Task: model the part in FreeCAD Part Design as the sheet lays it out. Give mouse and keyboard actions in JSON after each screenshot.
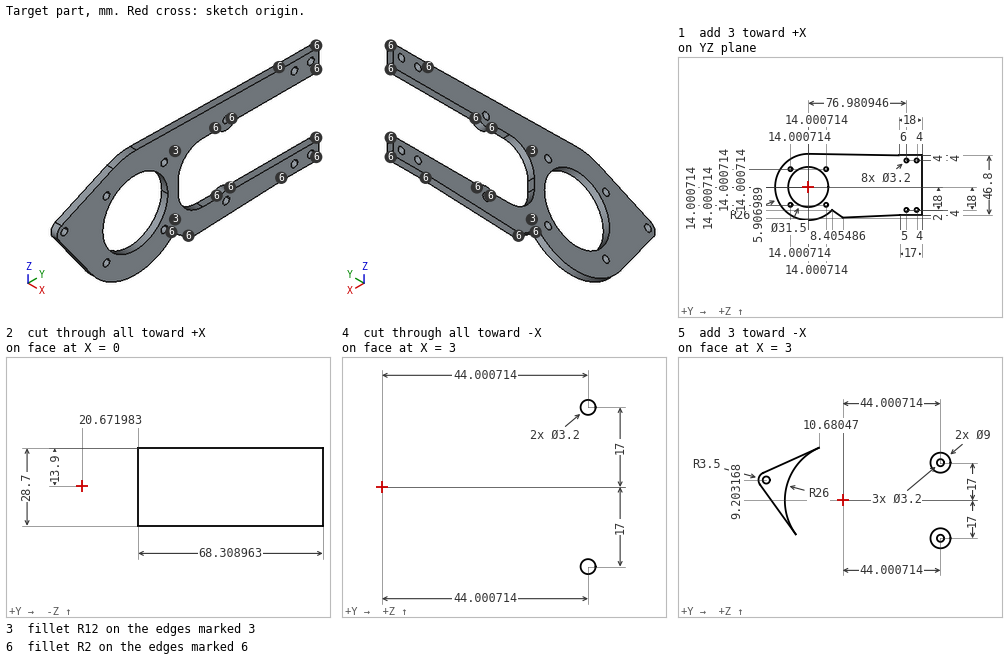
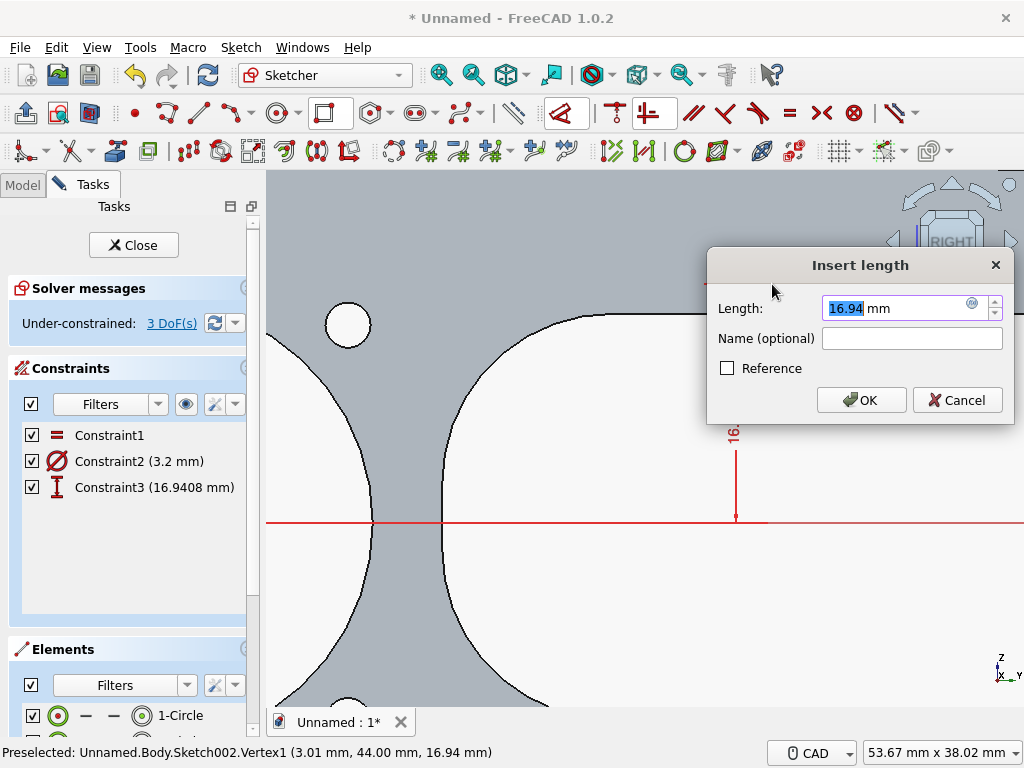
{"action": "type", "text": "17"}
{"action": "key", "text": "Return"}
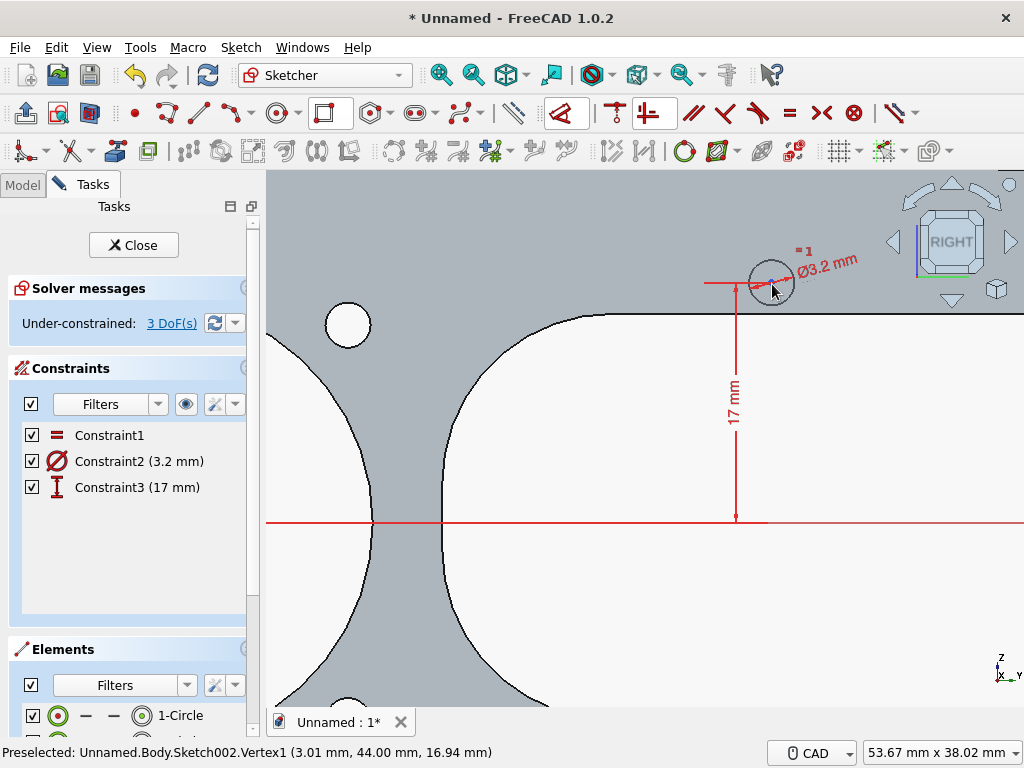
{"action": "scroll", "coordinate": [788, 267], "scroll_direction": "down", "scroll_amount": 2}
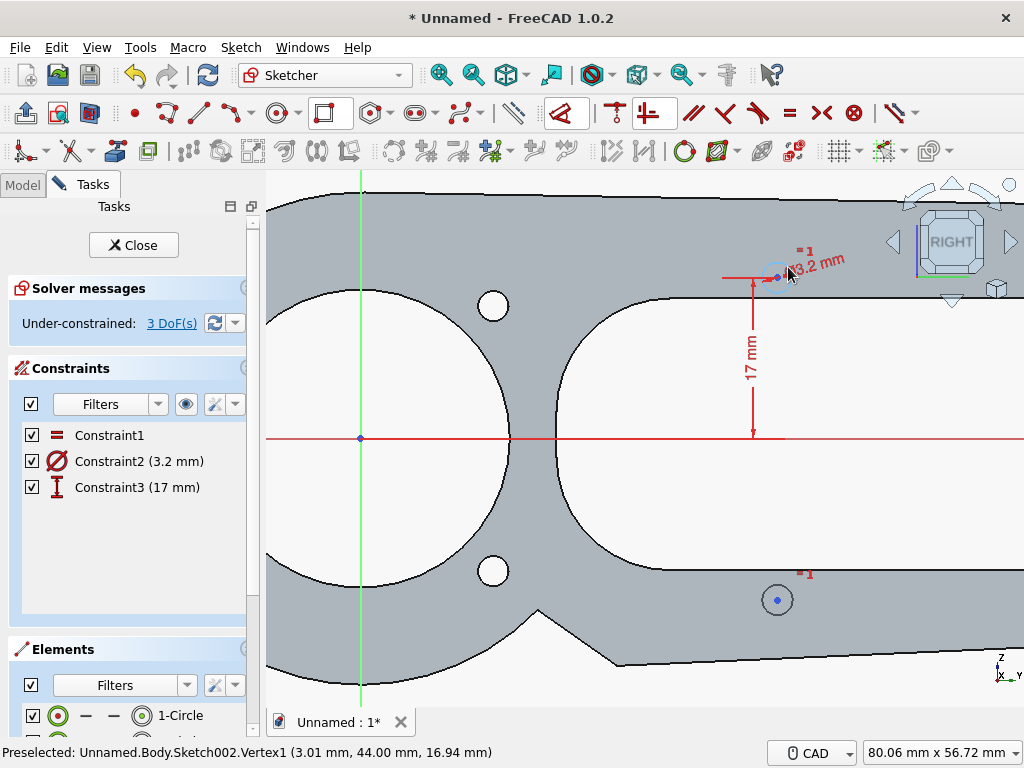
{"action": "left_click", "coordinate": [777, 600]}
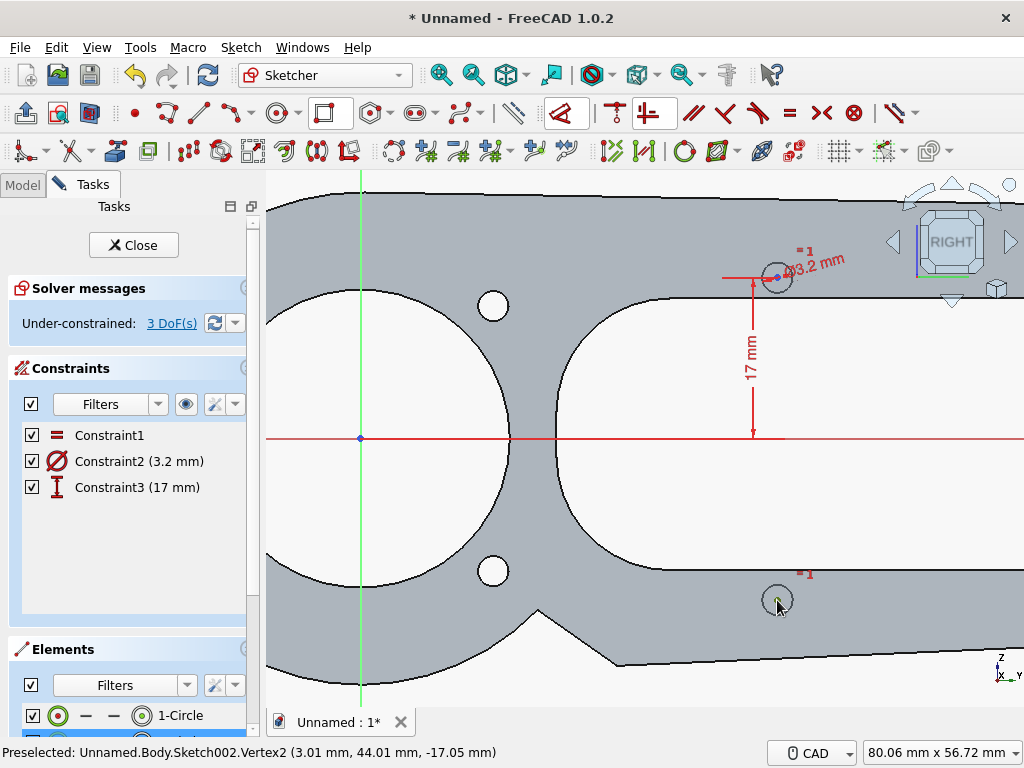
{"action": "left_click", "coordinate": [584, 114]}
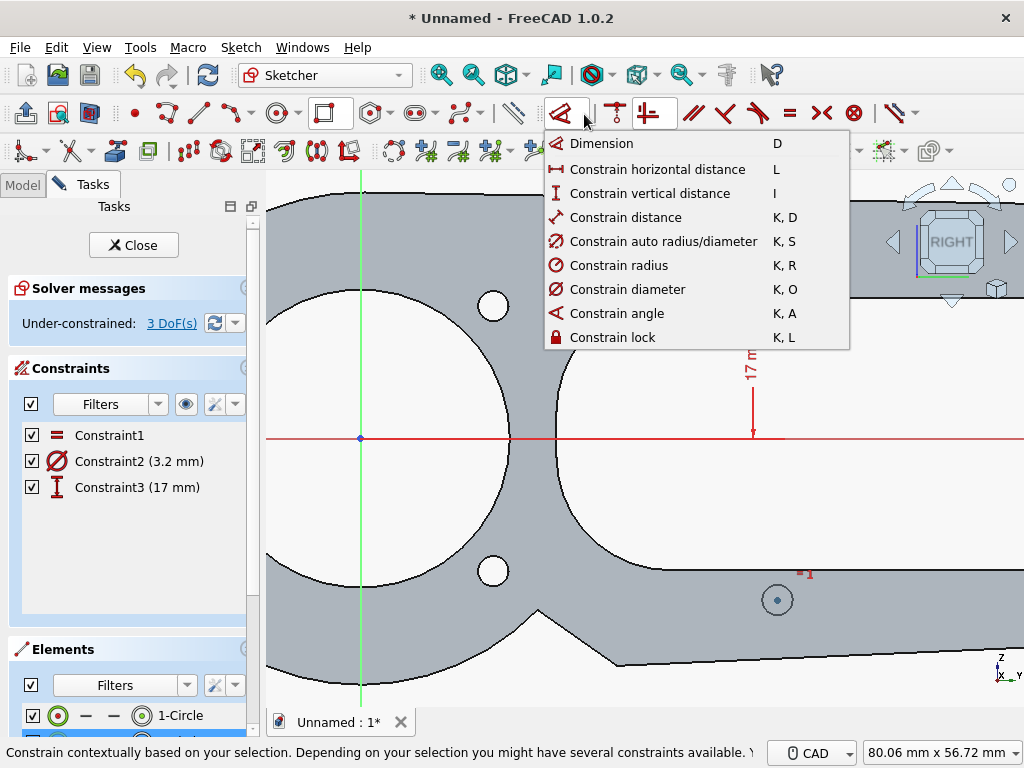
{"action": "left_click", "coordinate": [697, 193]}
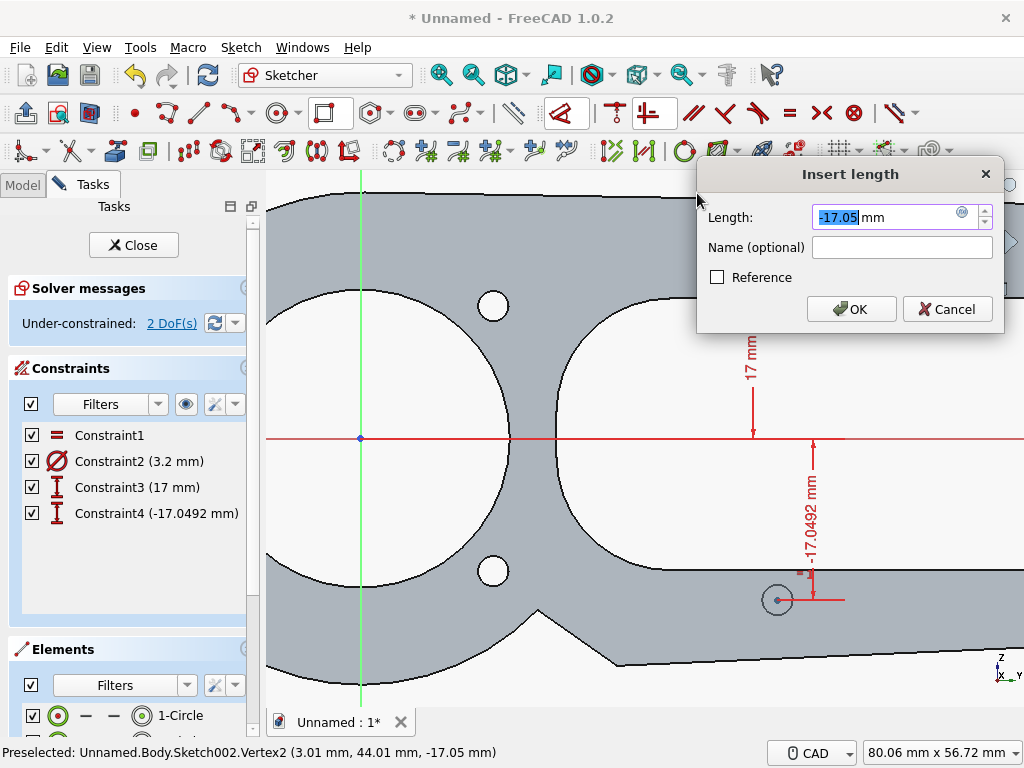
{"action": "type", "text": "-17"}
{"action": "key", "text": "Return"}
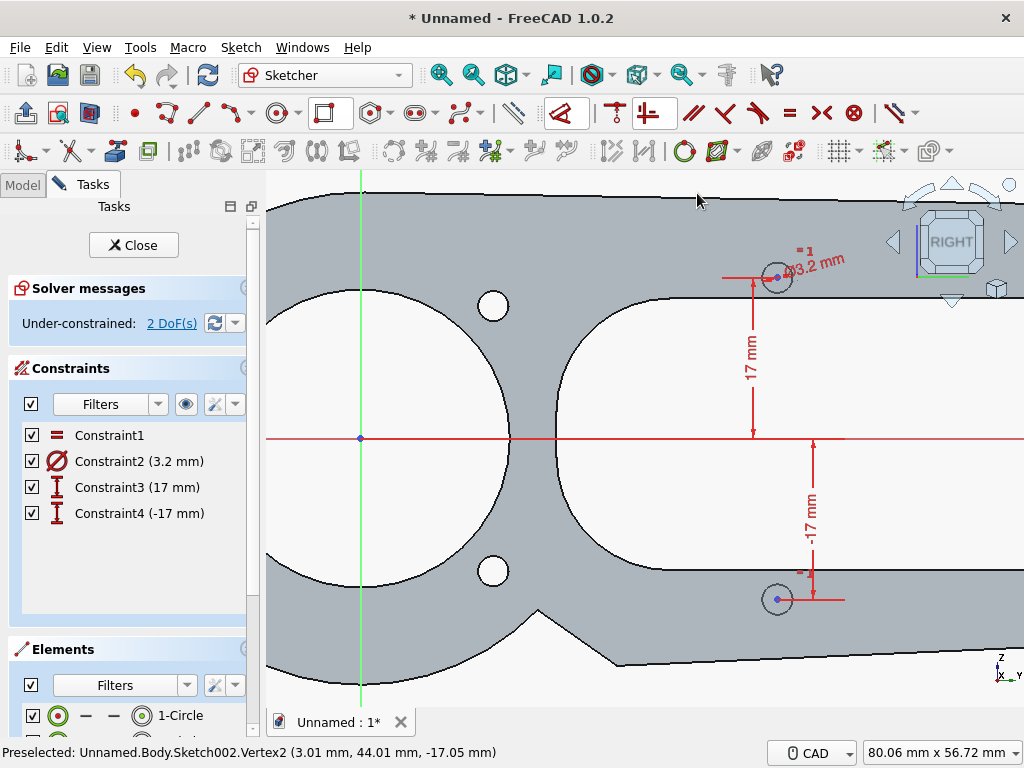
{"action": "left_click", "coordinate": [777, 278]}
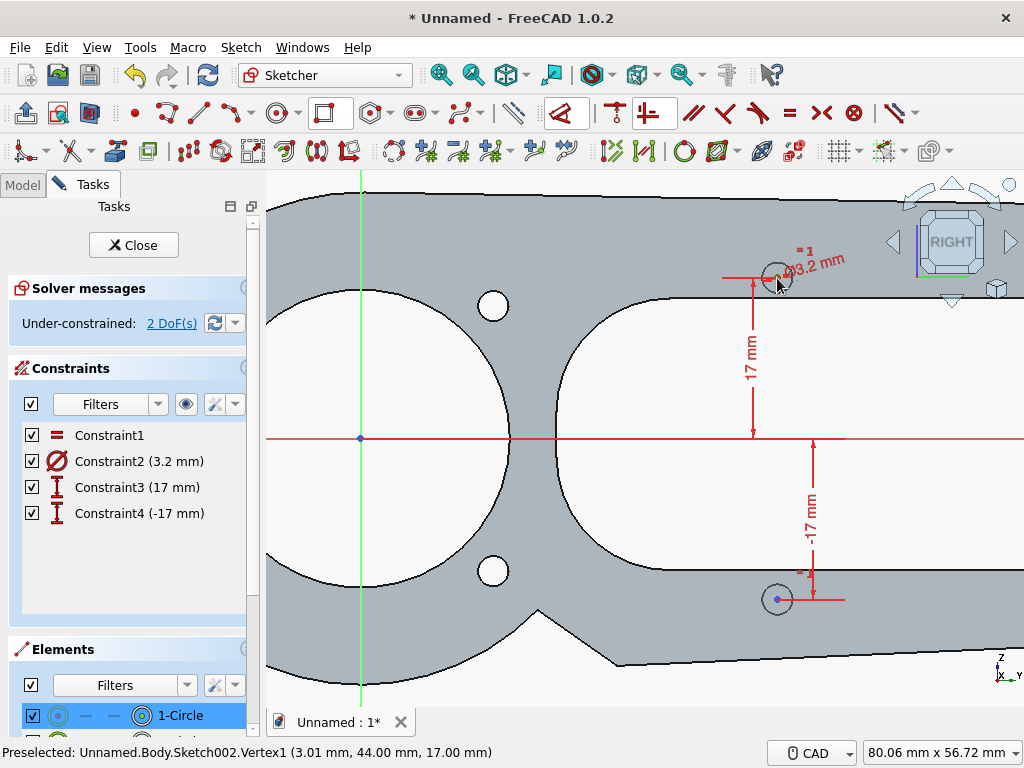
{"action": "key", "text": "l"}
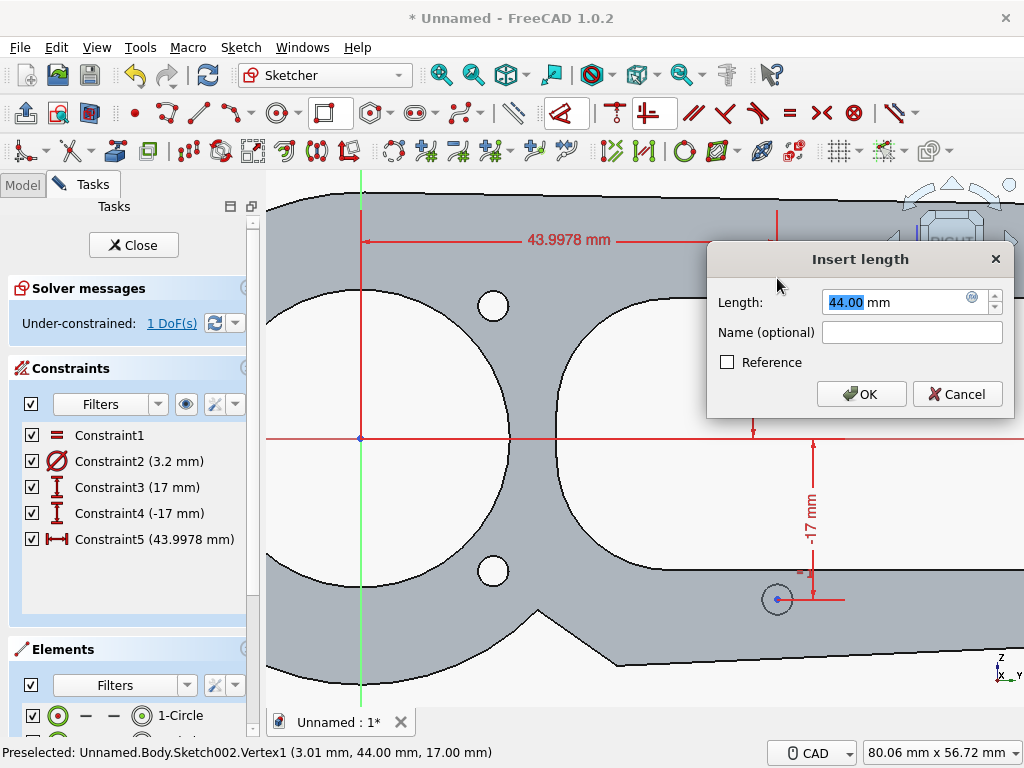
{"action": "type", "text": "44.000714"}
{"action": "key", "text": "Return"}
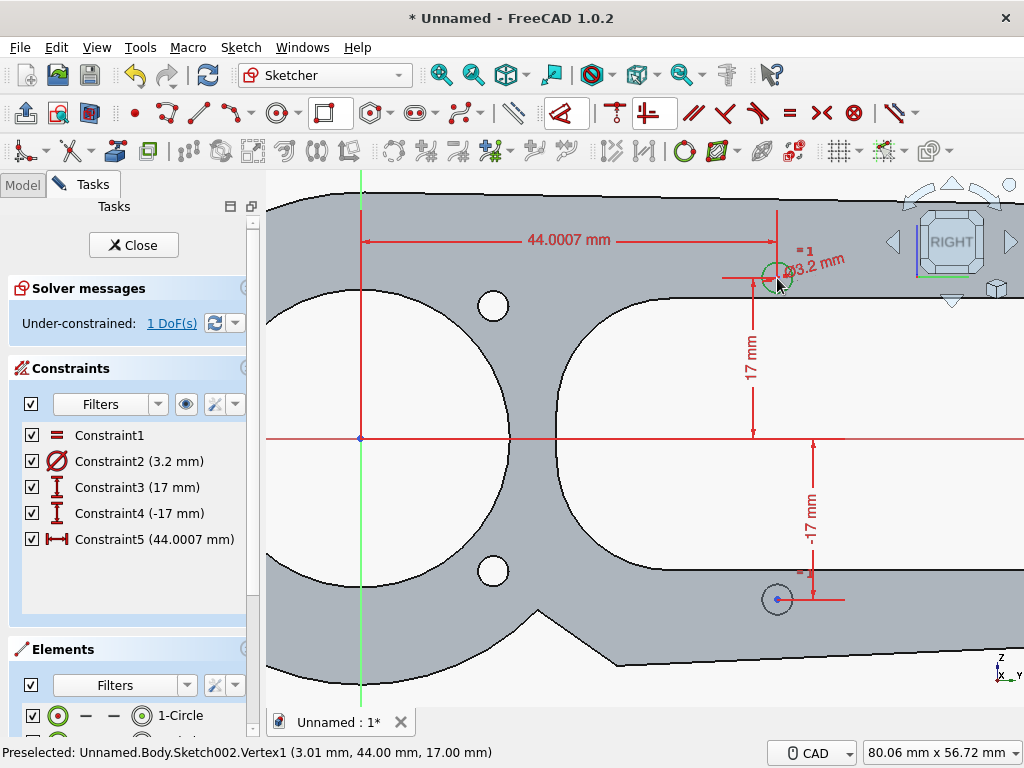
{"action": "left_click", "coordinate": [777, 600]}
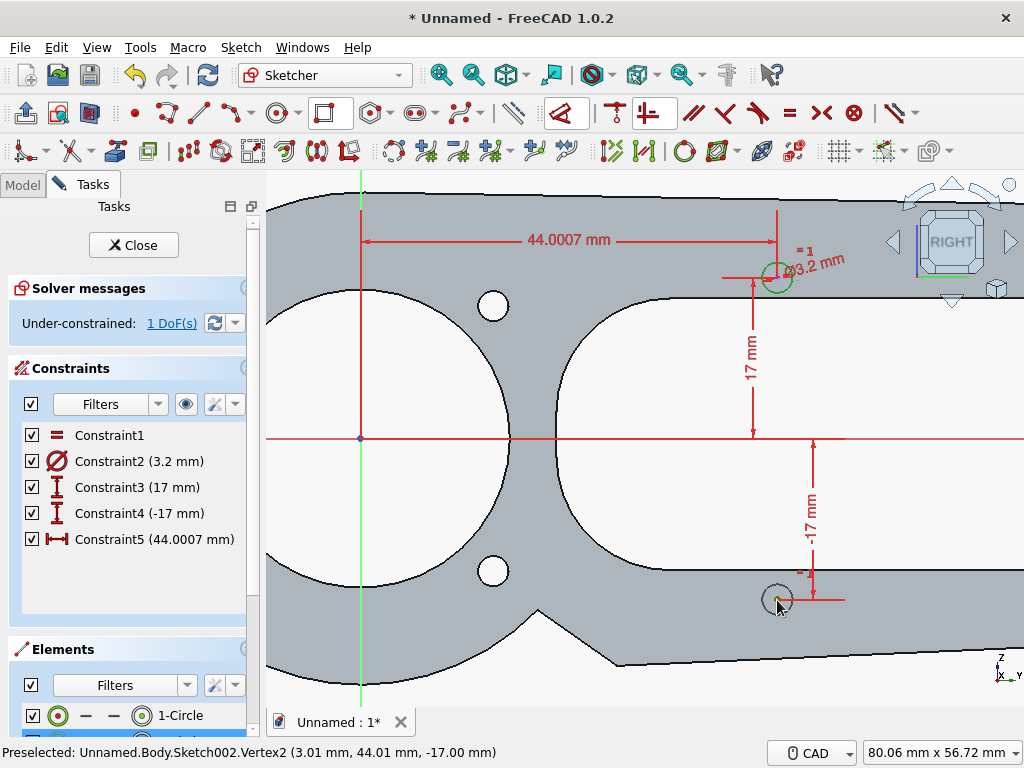
{"action": "left_click", "coordinate": [584, 114]}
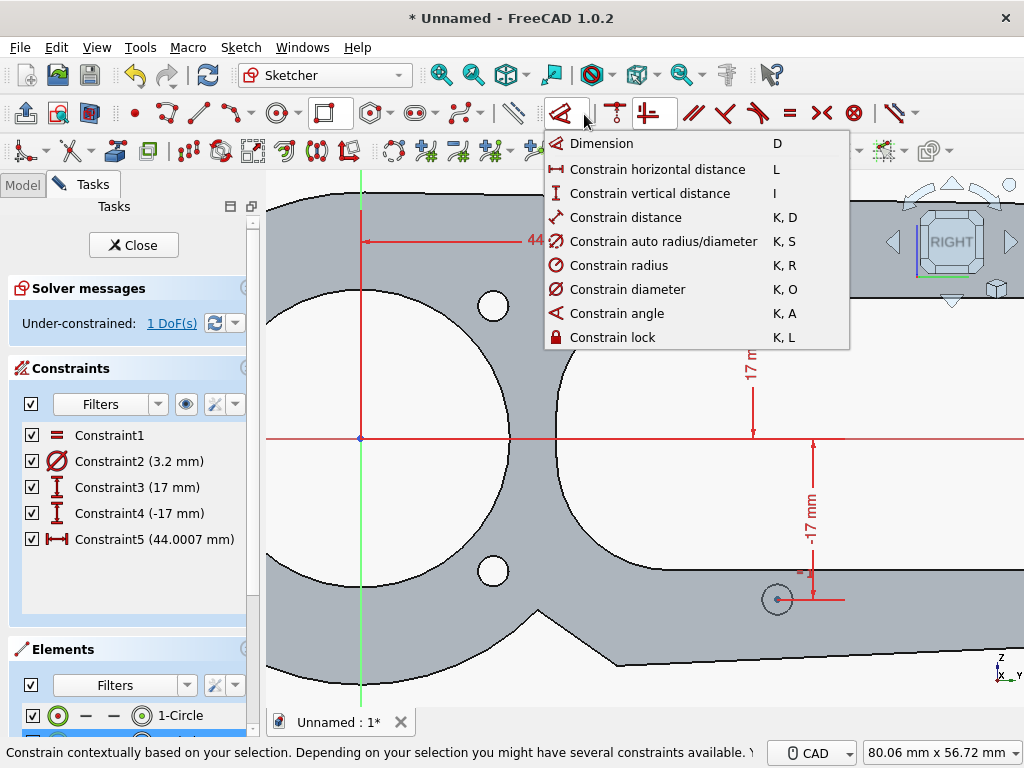
{"action": "left_click", "coordinate": [697, 169]}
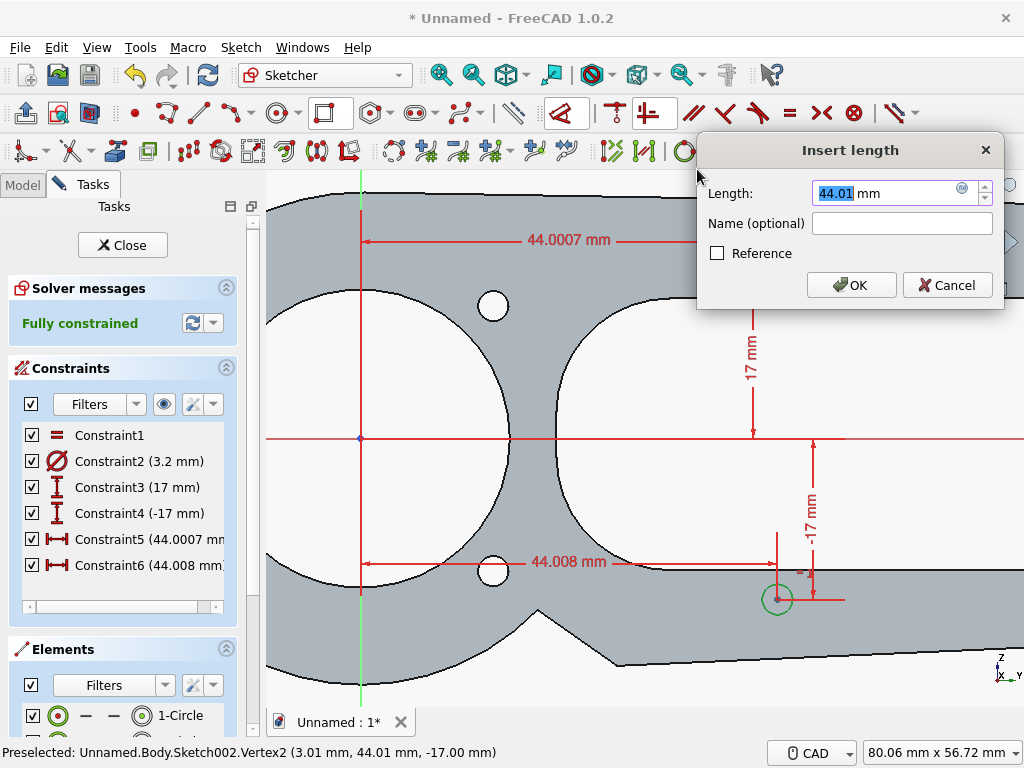
{"action": "type", "text": "44.000714"}
{"action": "key", "text": "Return"}